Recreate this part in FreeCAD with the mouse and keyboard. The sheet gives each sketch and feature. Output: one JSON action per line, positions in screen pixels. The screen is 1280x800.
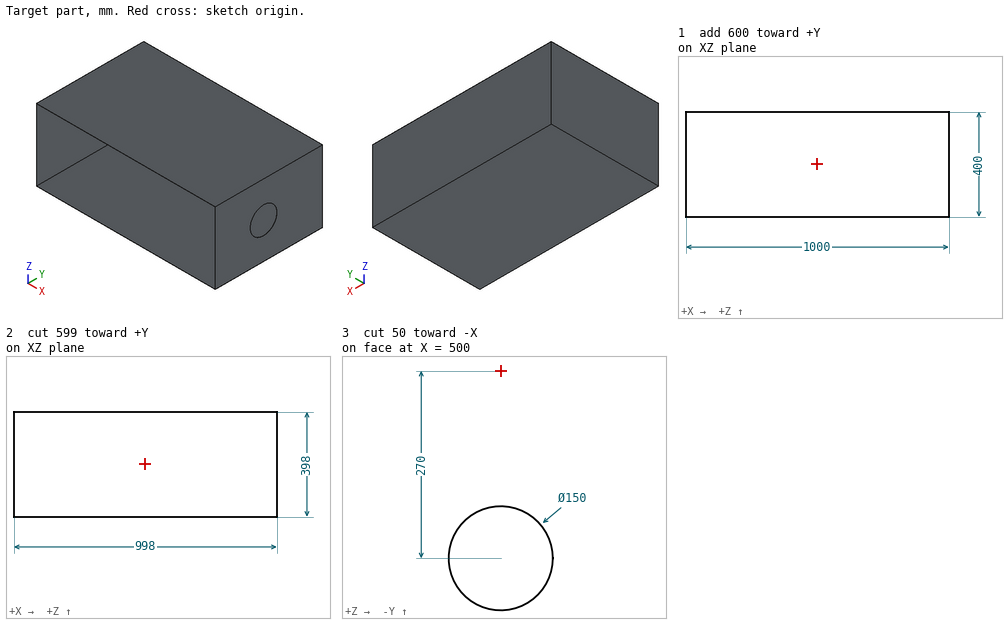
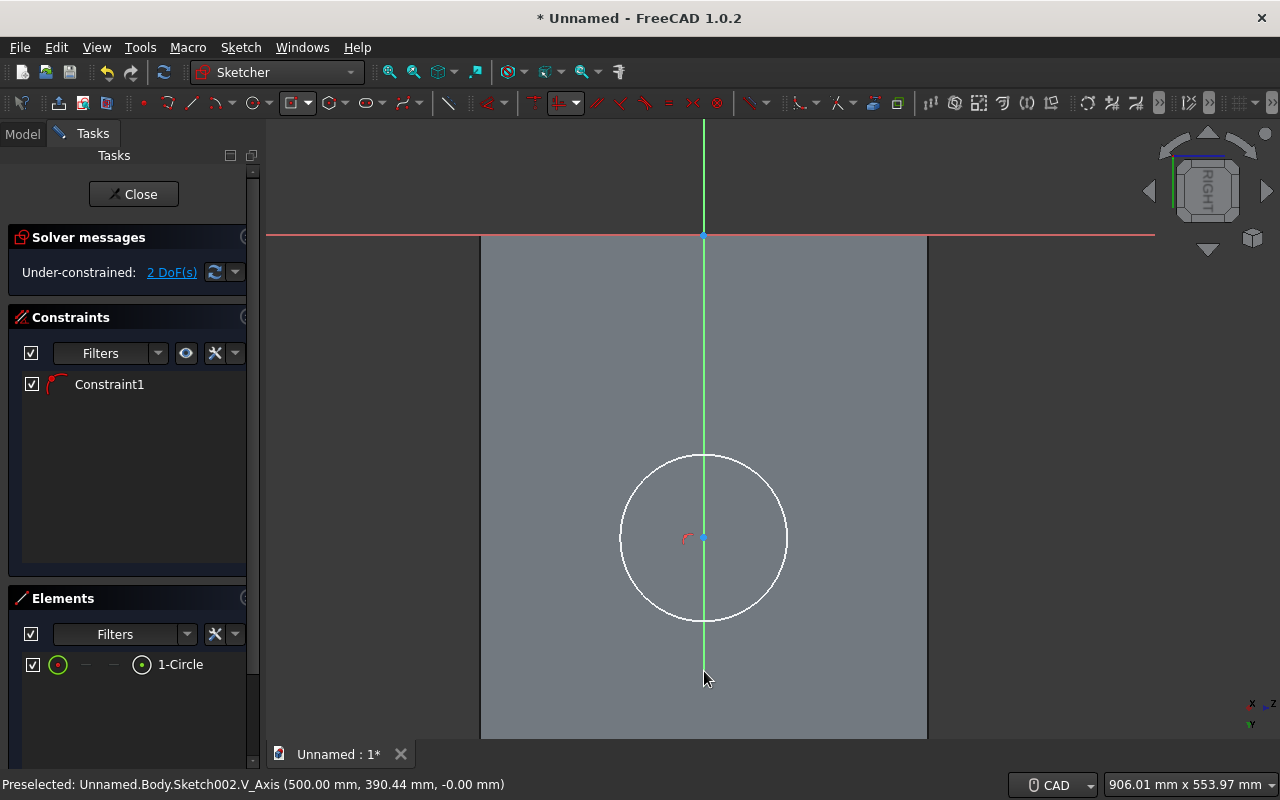
{"action": "key", "text": "d"}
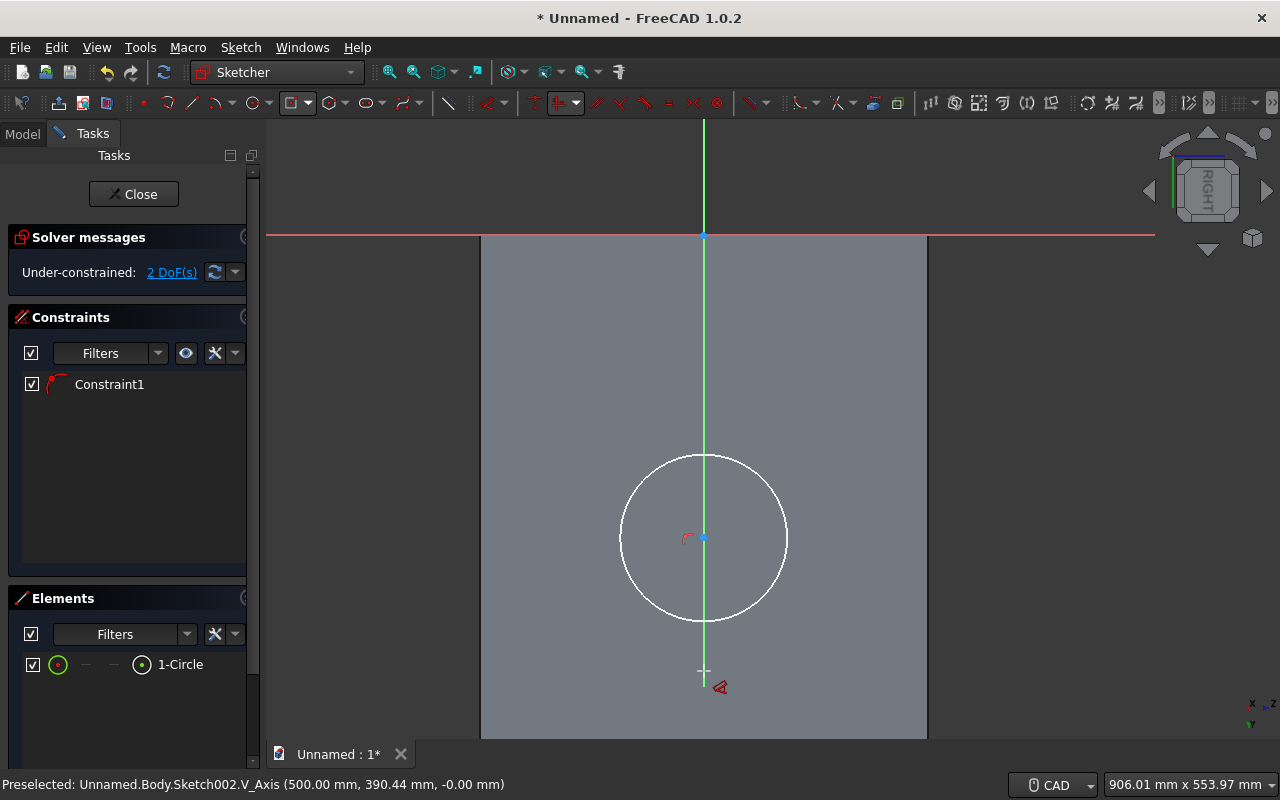
{"action": "left_click", "coordinate": [763, 479]}
{"action": "left_click", "coordinate": [786, 456]}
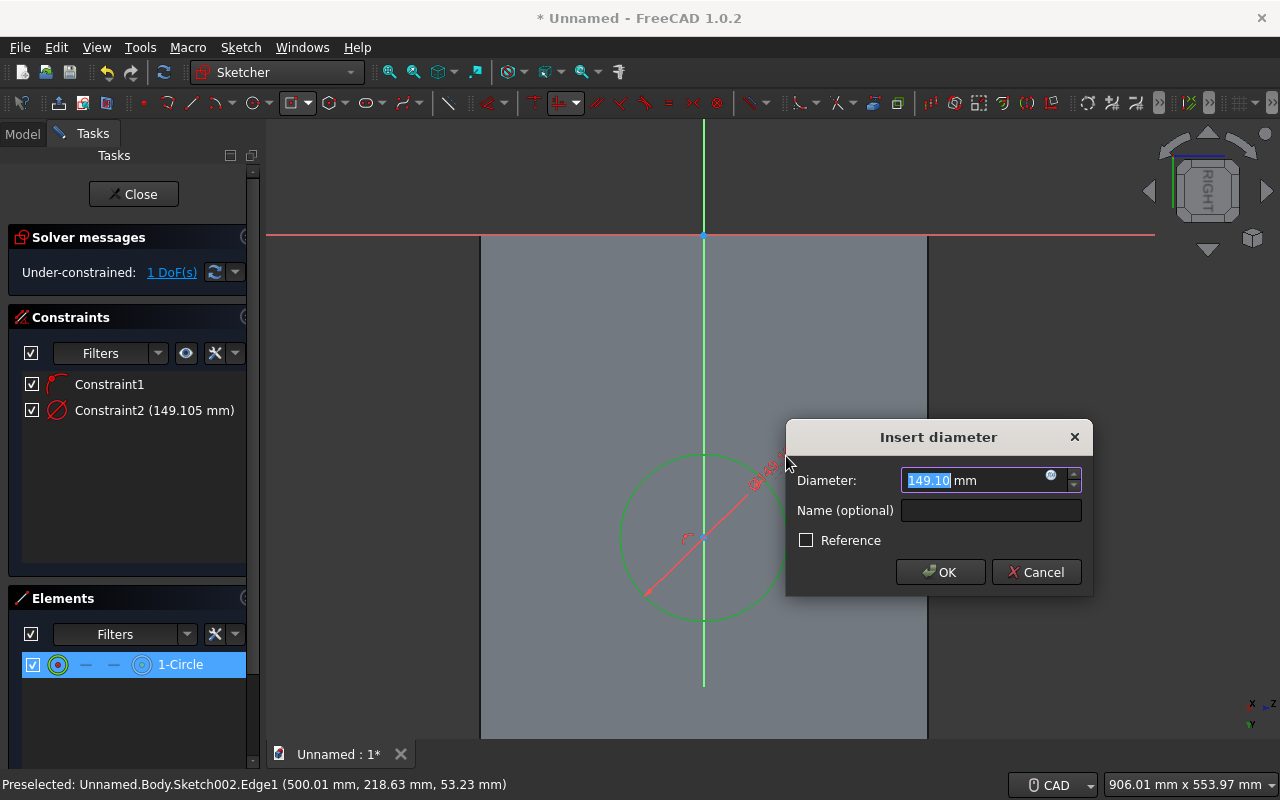
{"action": "type", "text": "150"}
{"action": "key", "text": "Return"}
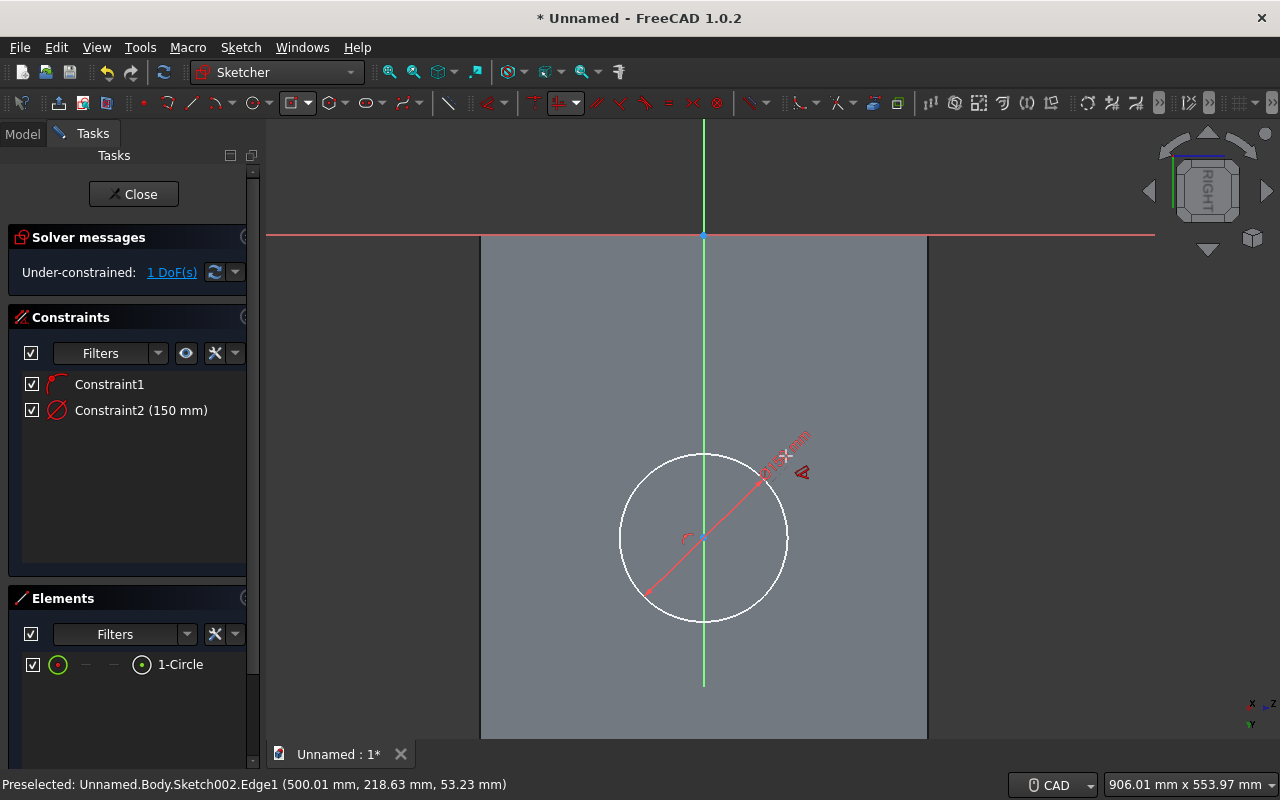
{"action": "left_click", "coordinate": [704, 538]}
{"action": "left_click", "coordinate": [738, 387]}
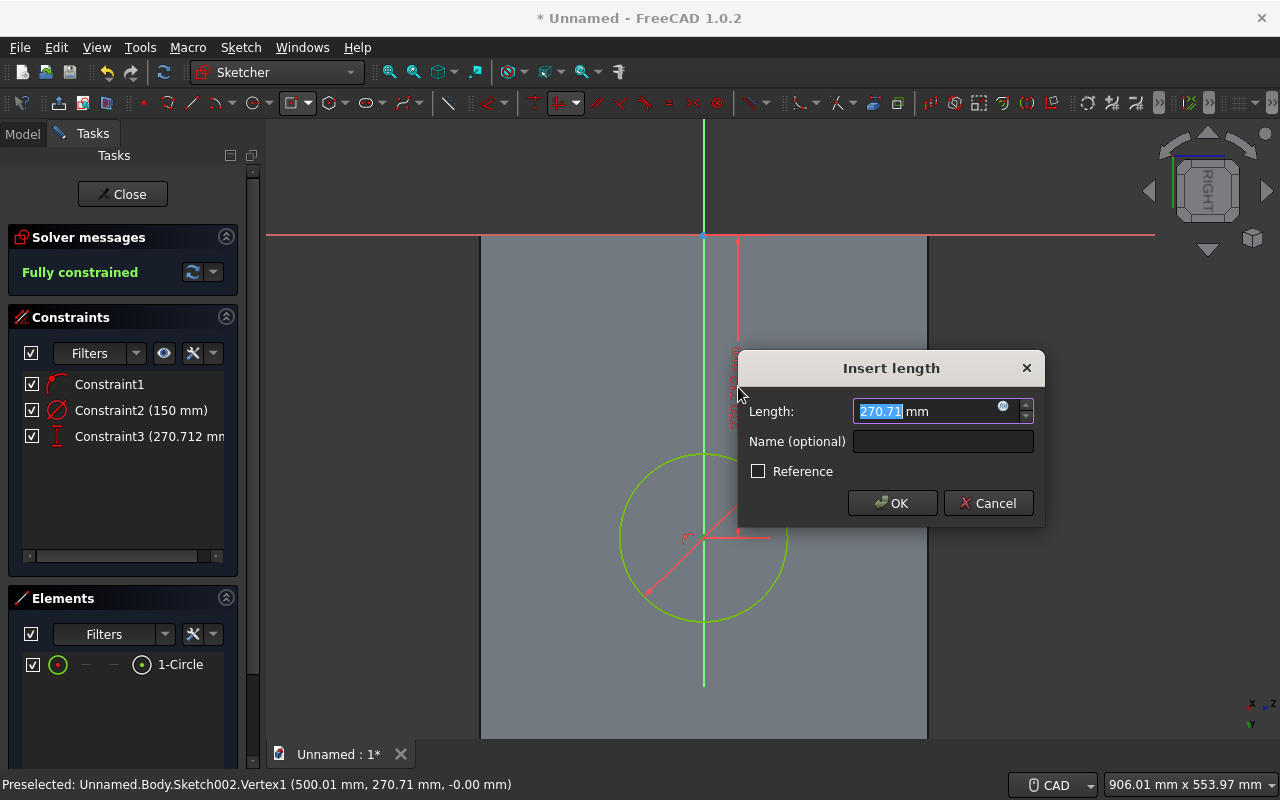
{"action": "type", "text": "270"}
{"action": "key", "text": "Return"}
{"action": "key", "text": "Escape"}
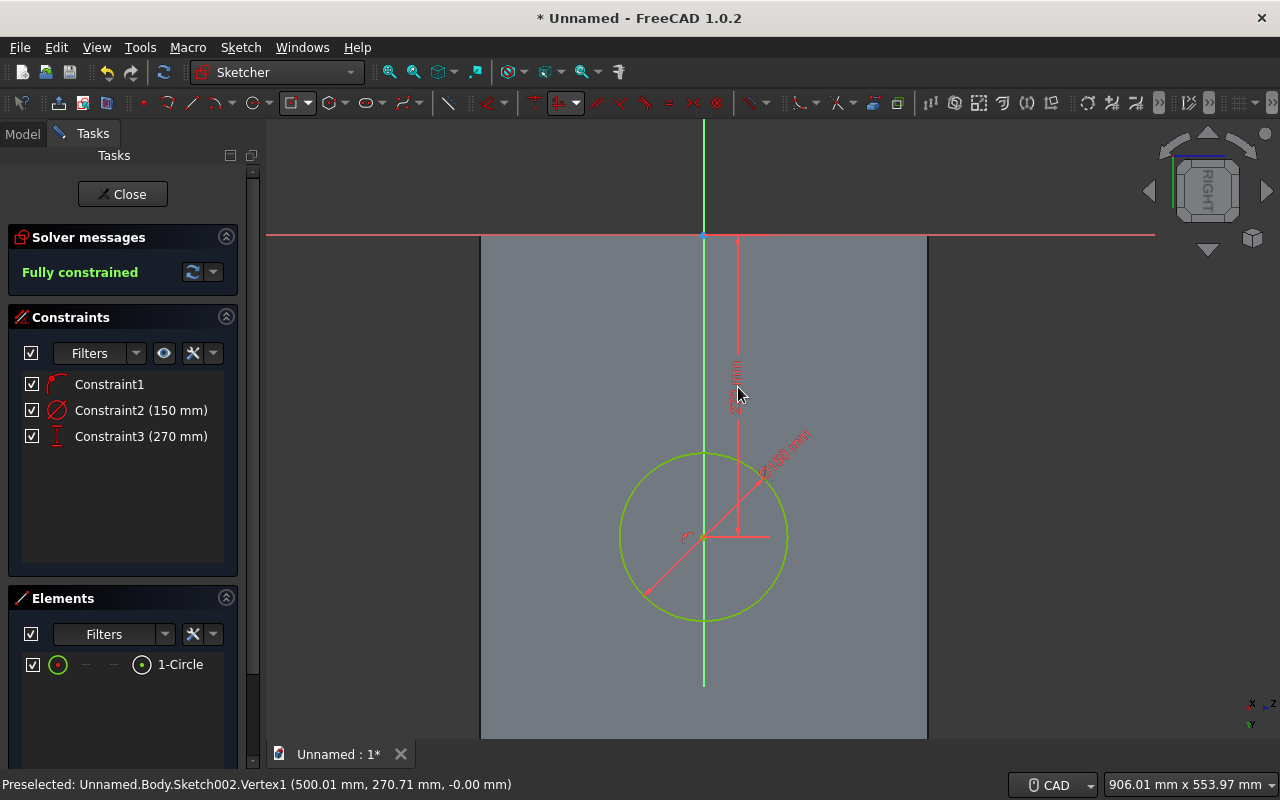
{"action": "left_click", "coordinate": [123, 194]}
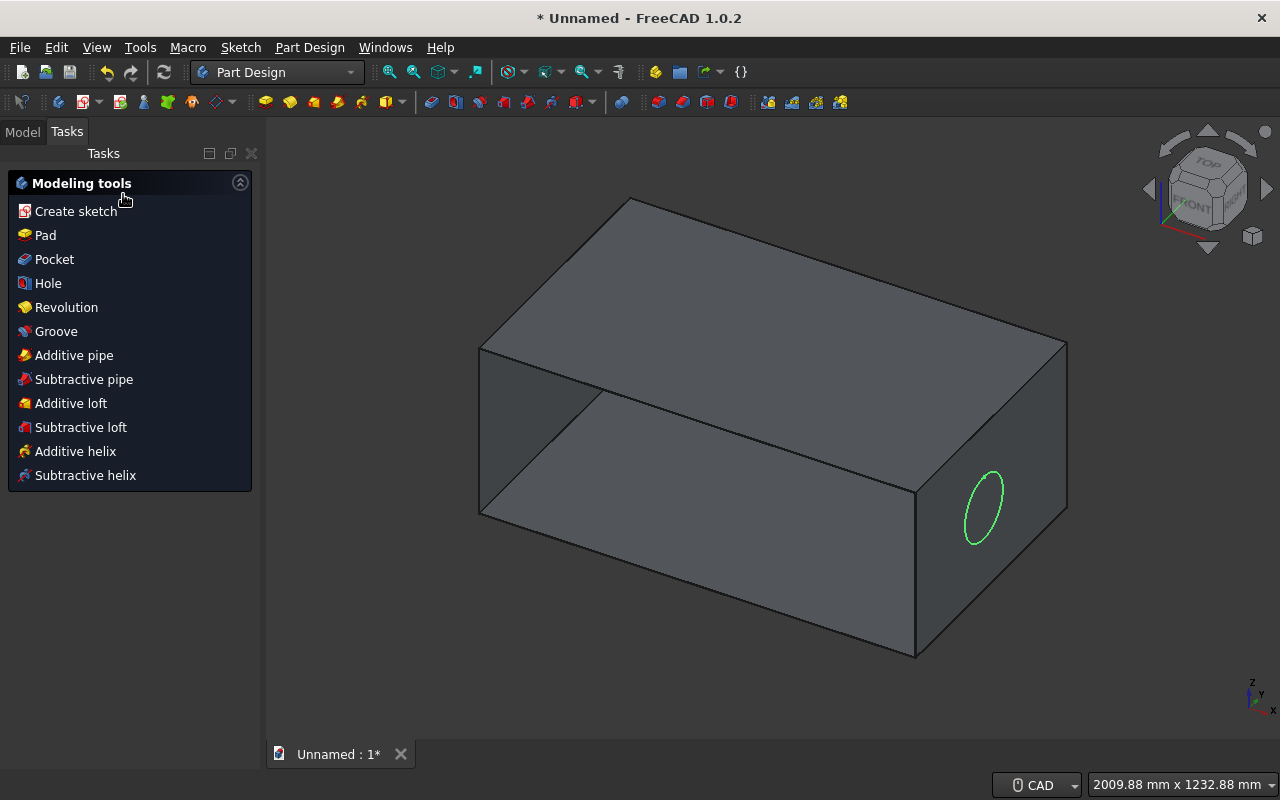
{"action": "left_click", "coordinate": [432, 102]}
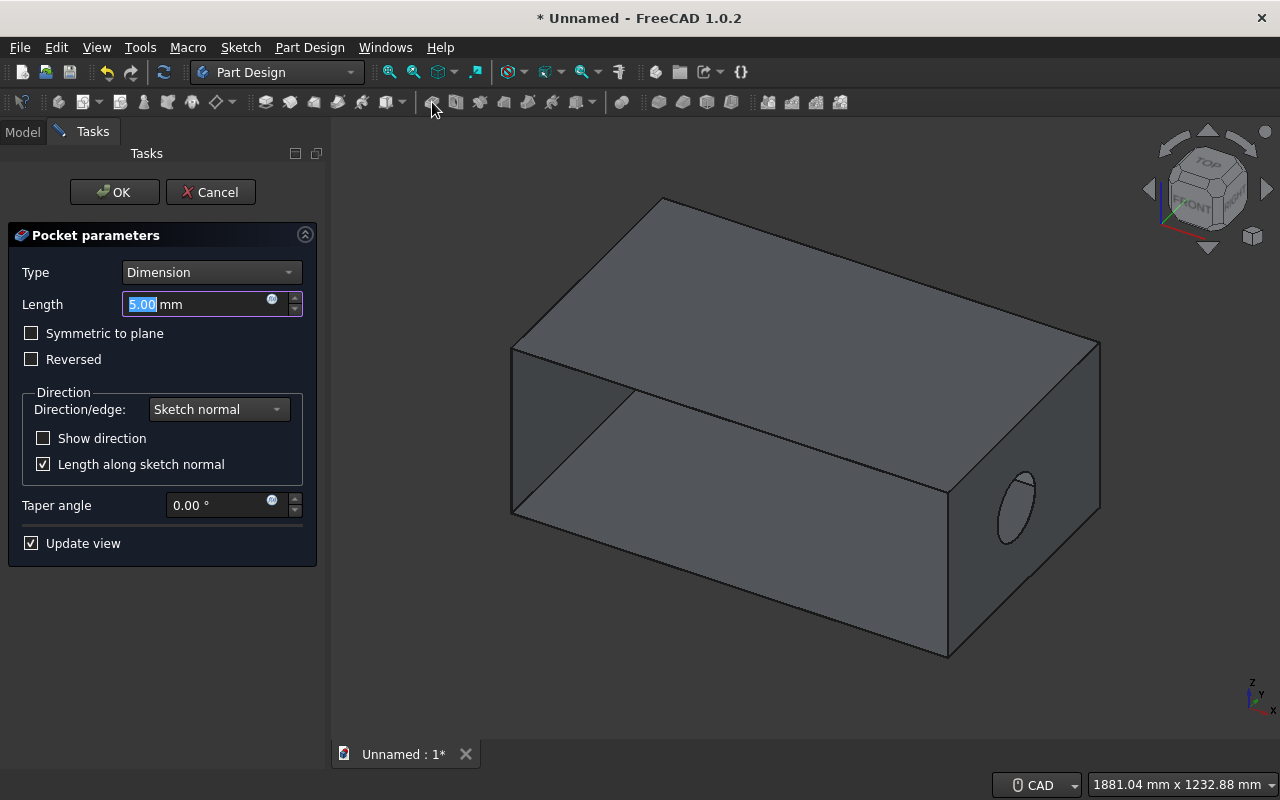
{"action": "type", "text": "50"}
{"action": "key", "text": "Tab"}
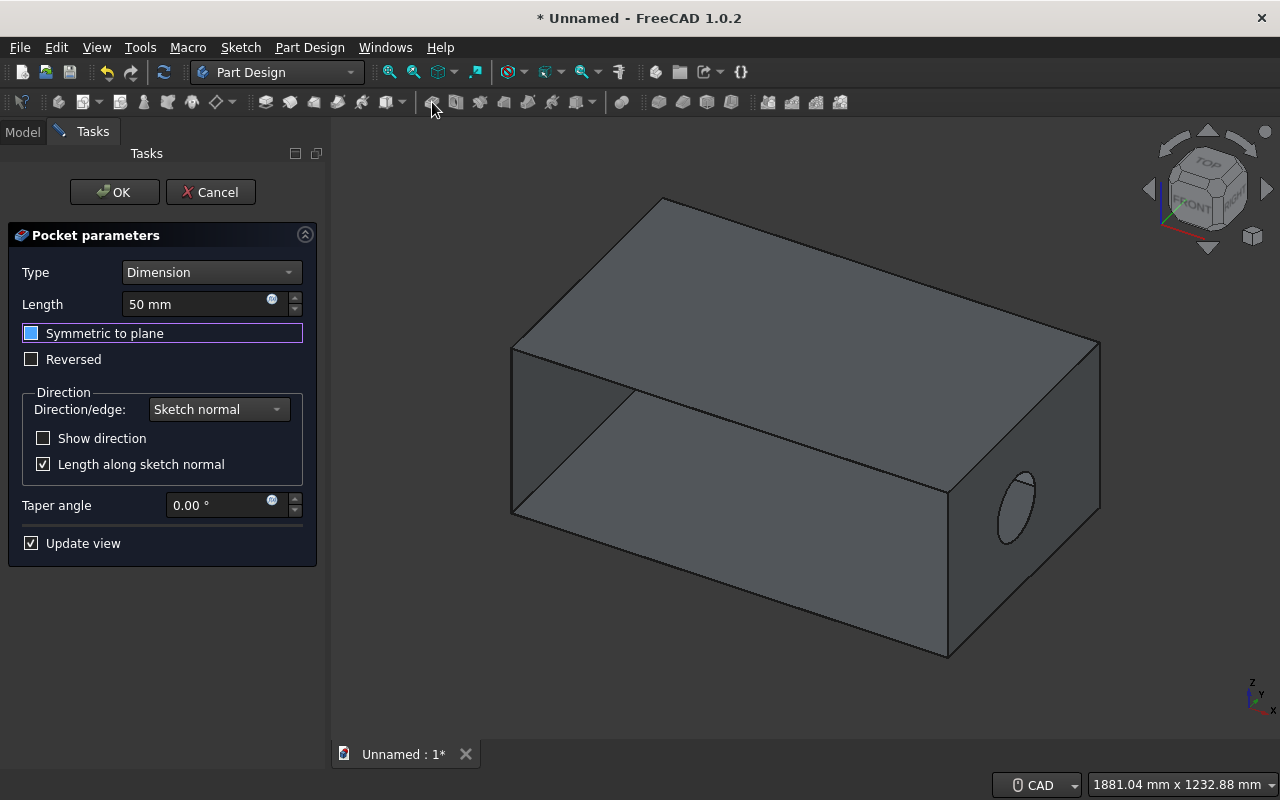
{"action": "left_click", "coordinate": [115, 192]}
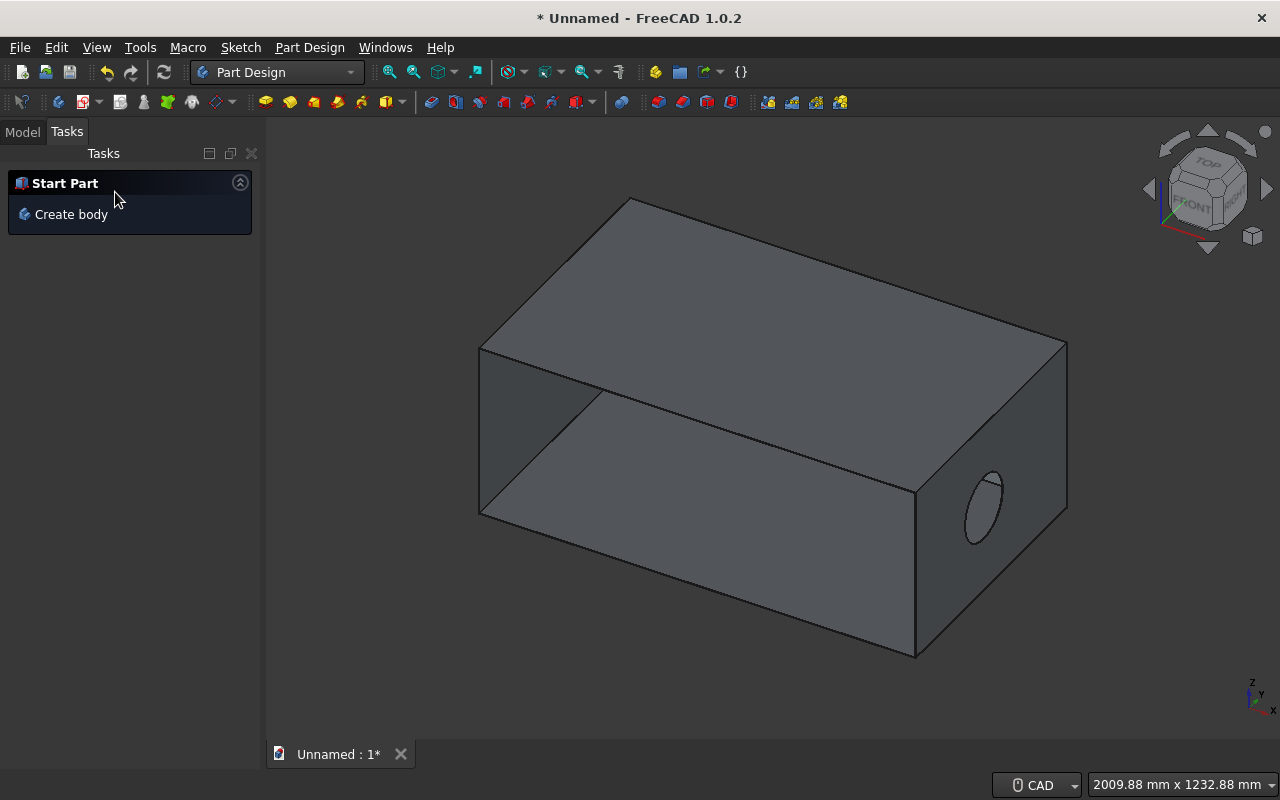
{"action": "key", "text": "0"}